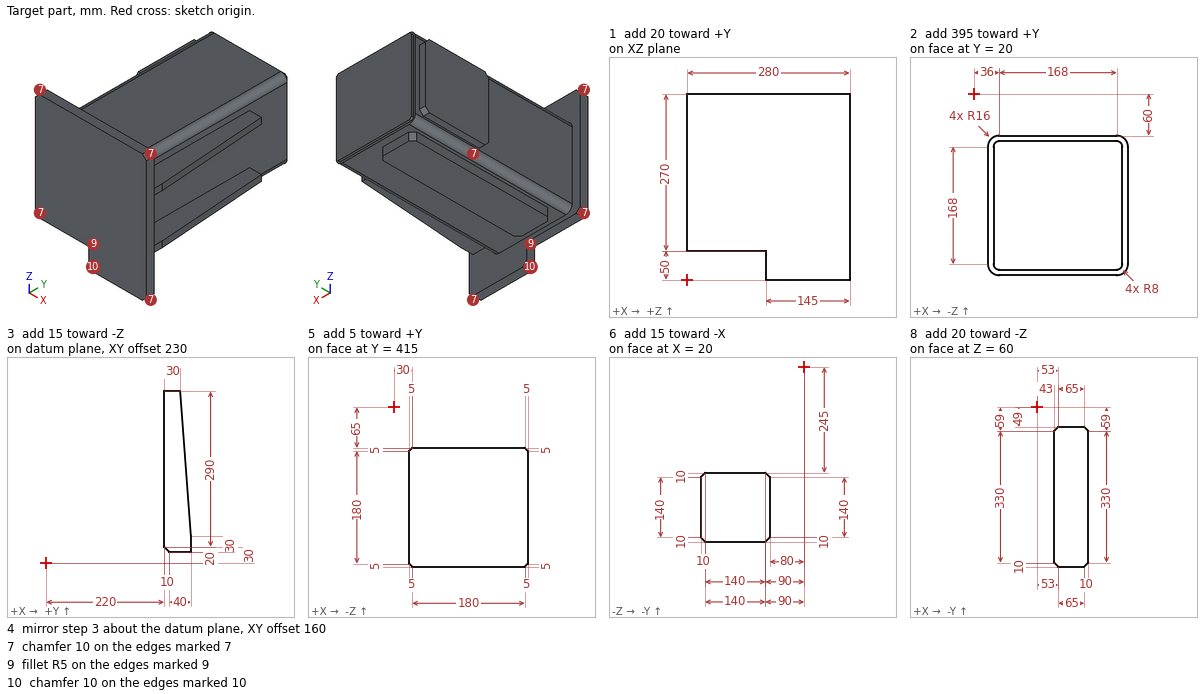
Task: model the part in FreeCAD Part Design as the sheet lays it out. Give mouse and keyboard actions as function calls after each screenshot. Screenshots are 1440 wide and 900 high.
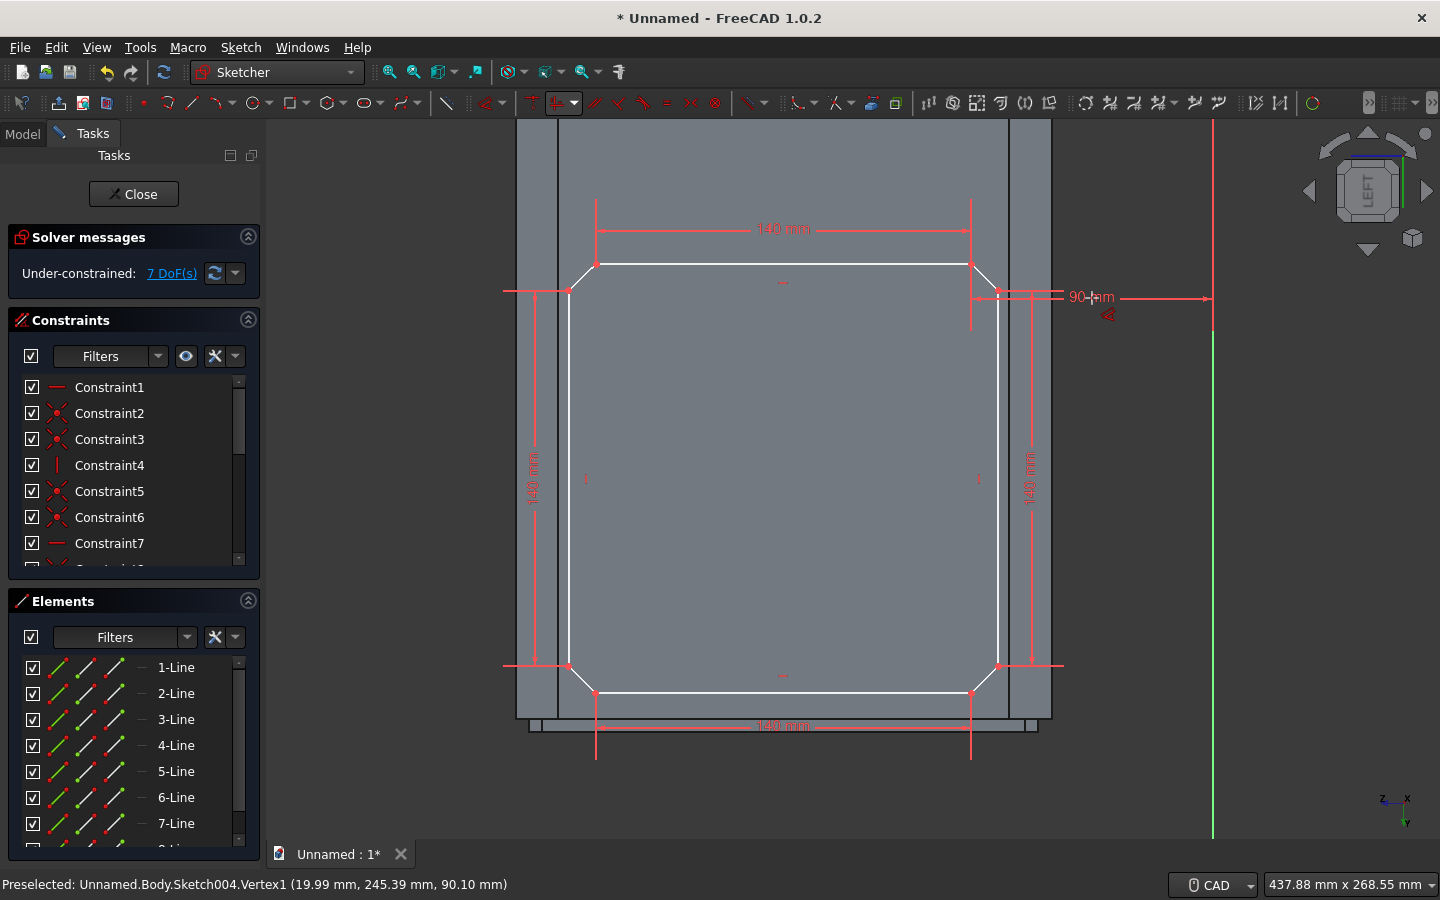
click(971, 693)
click(1092, 727)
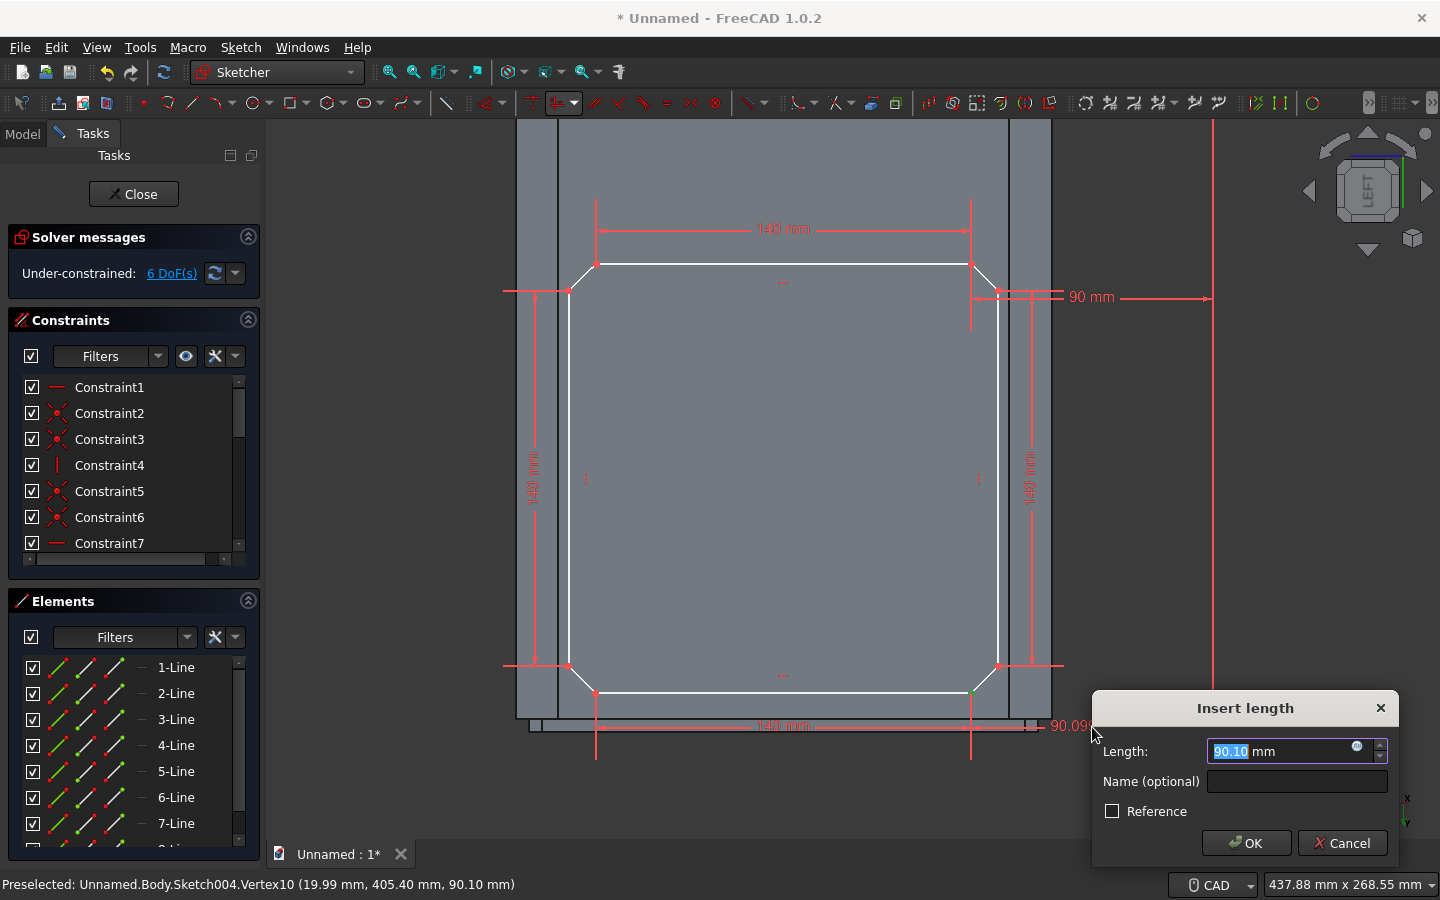
text(90)
key(Return)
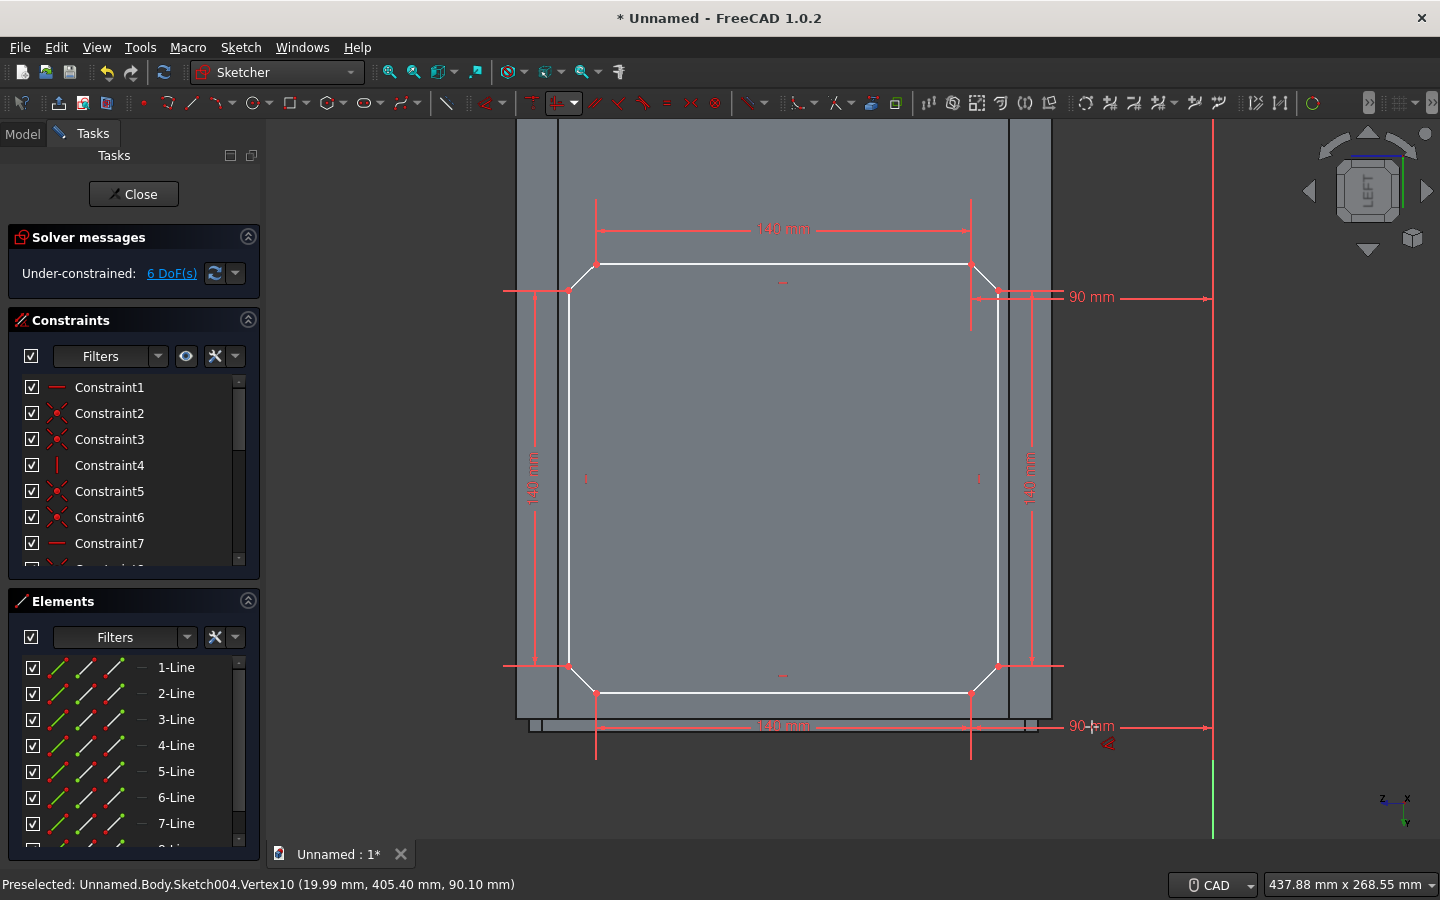
click(998, 666)
click(1105, 700)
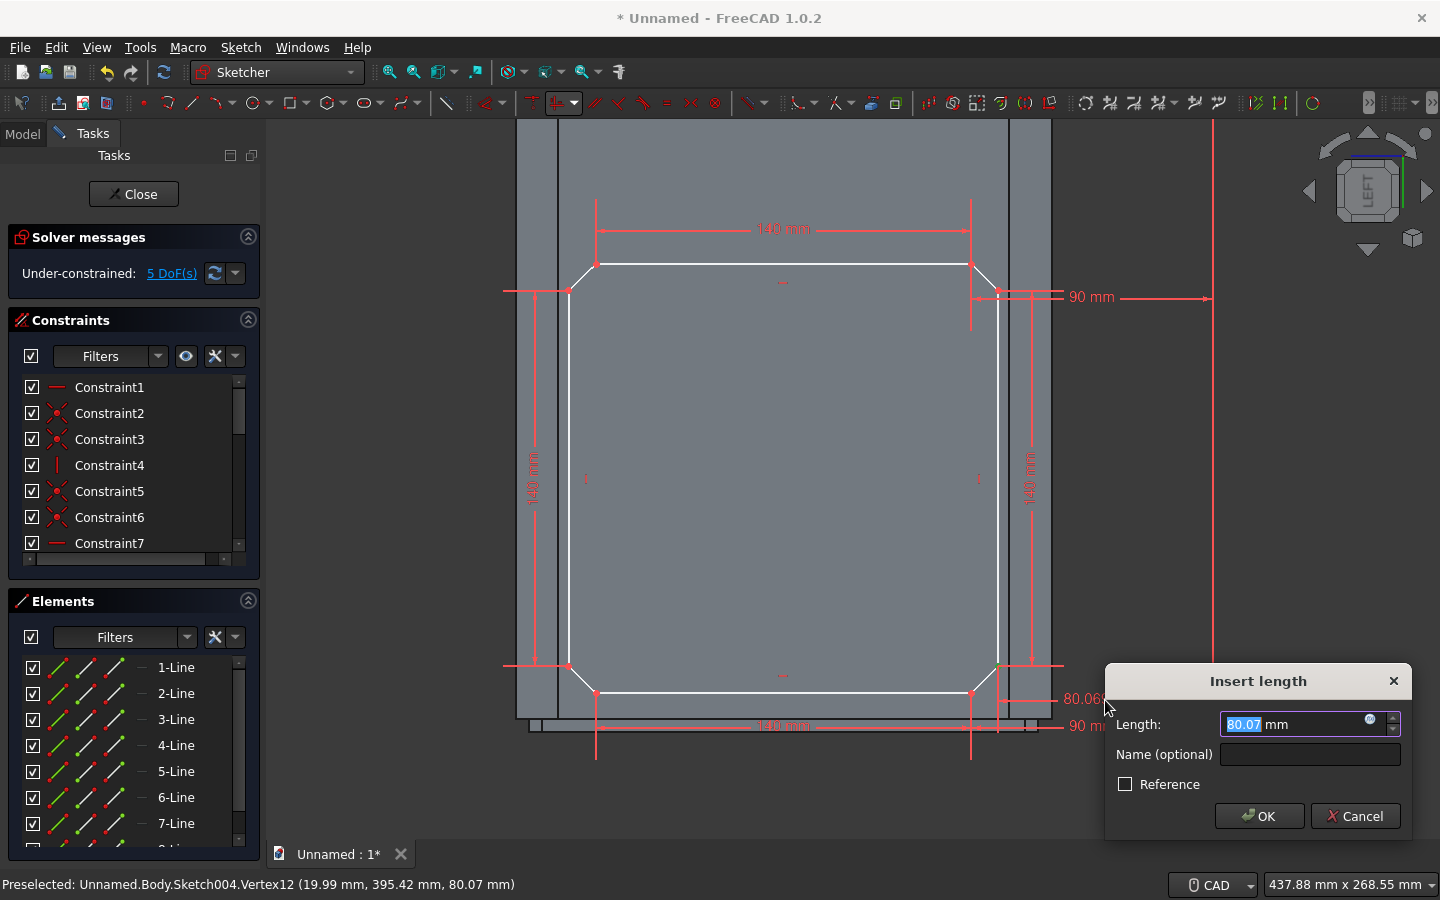
text(80)
key(Return)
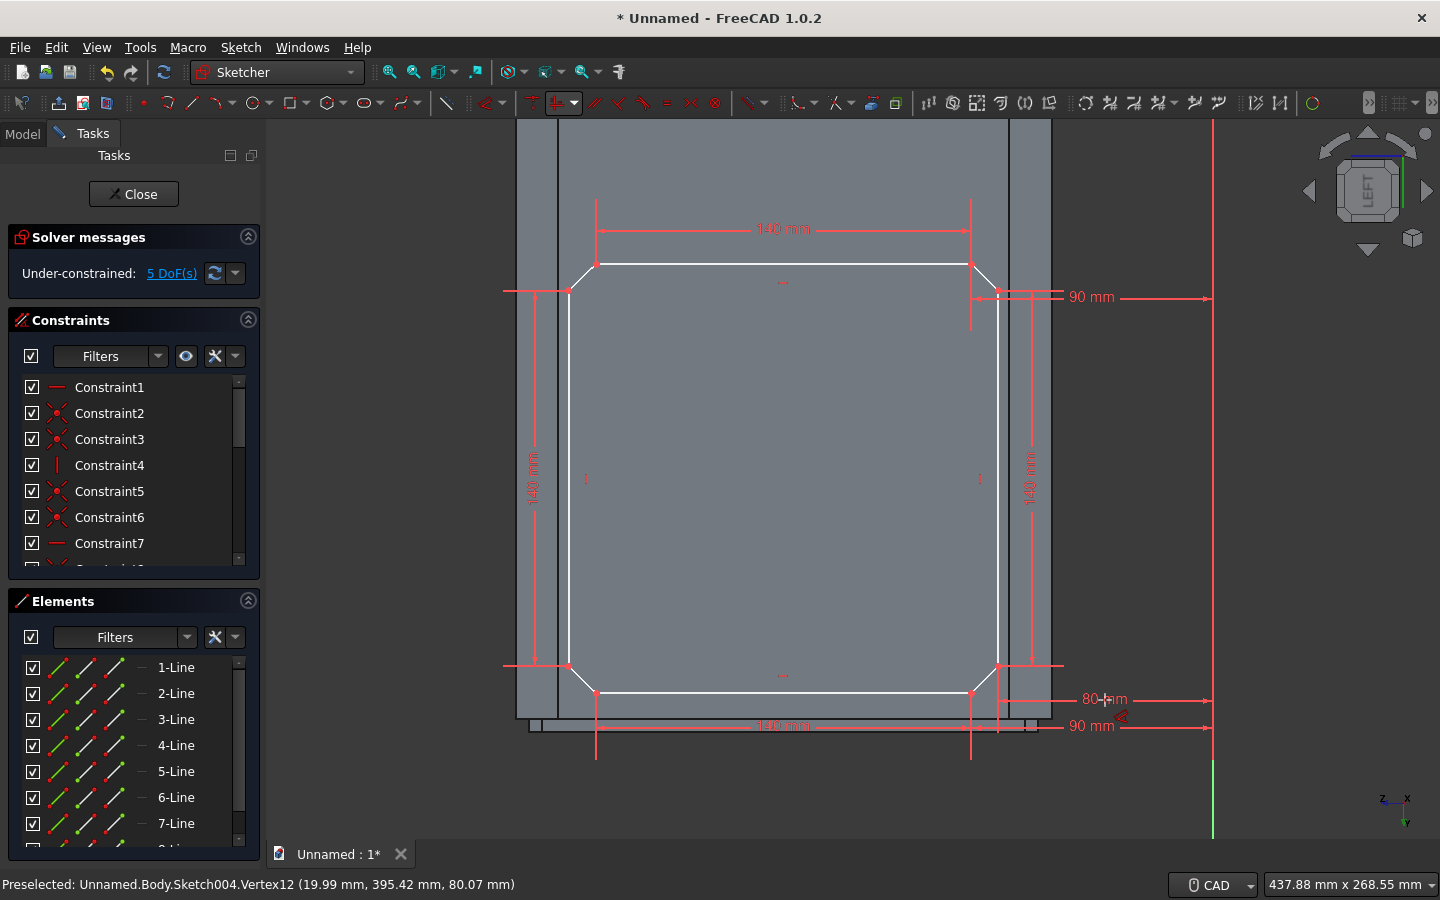
scroll(588, 272, up, 2)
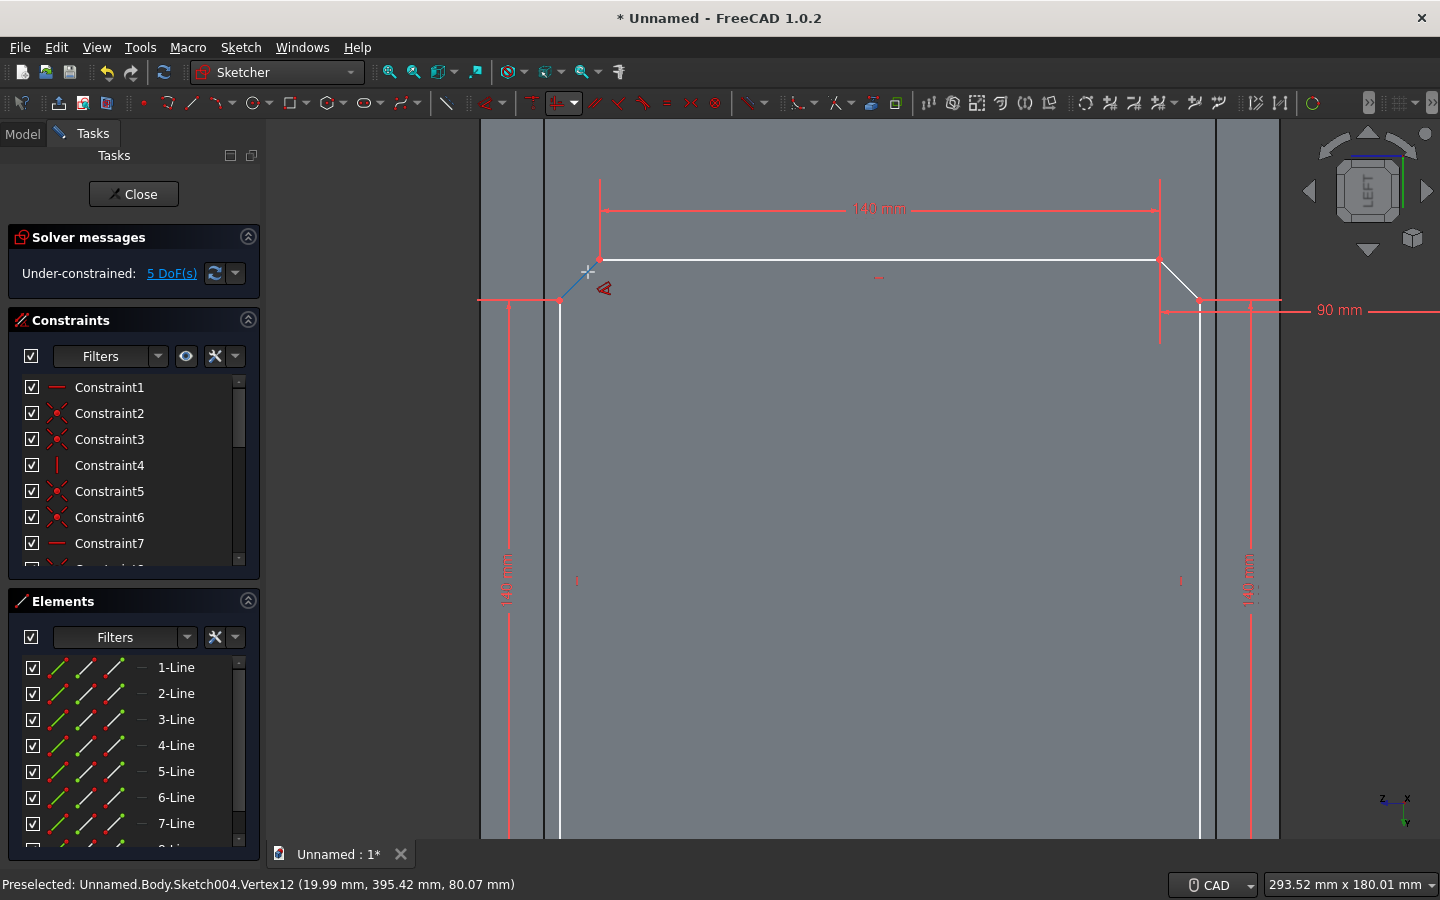
click(588, 272)
click(580, 226)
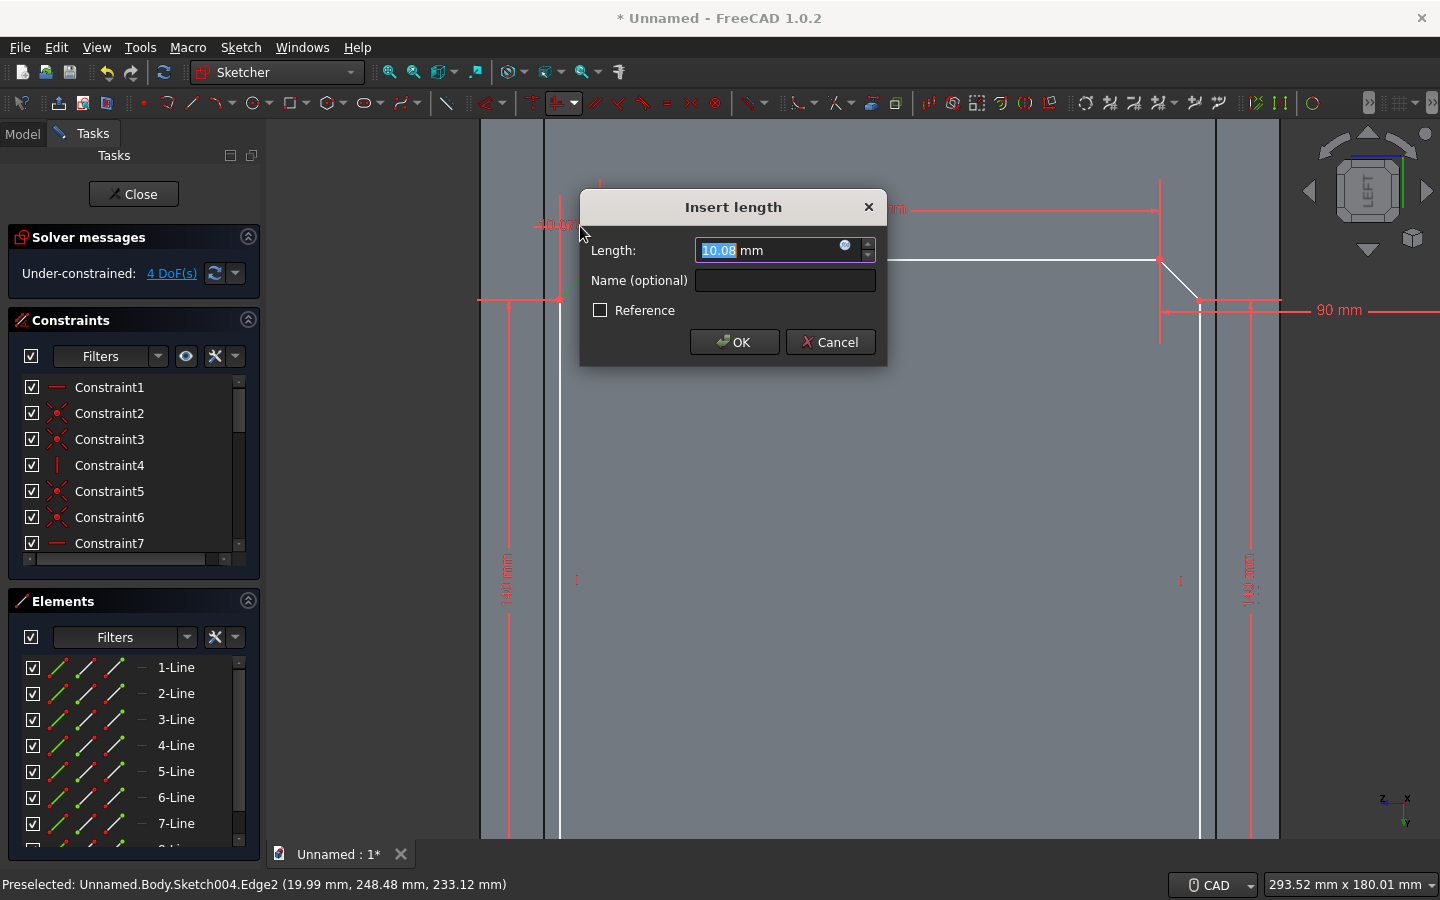
text(10)
key(Return)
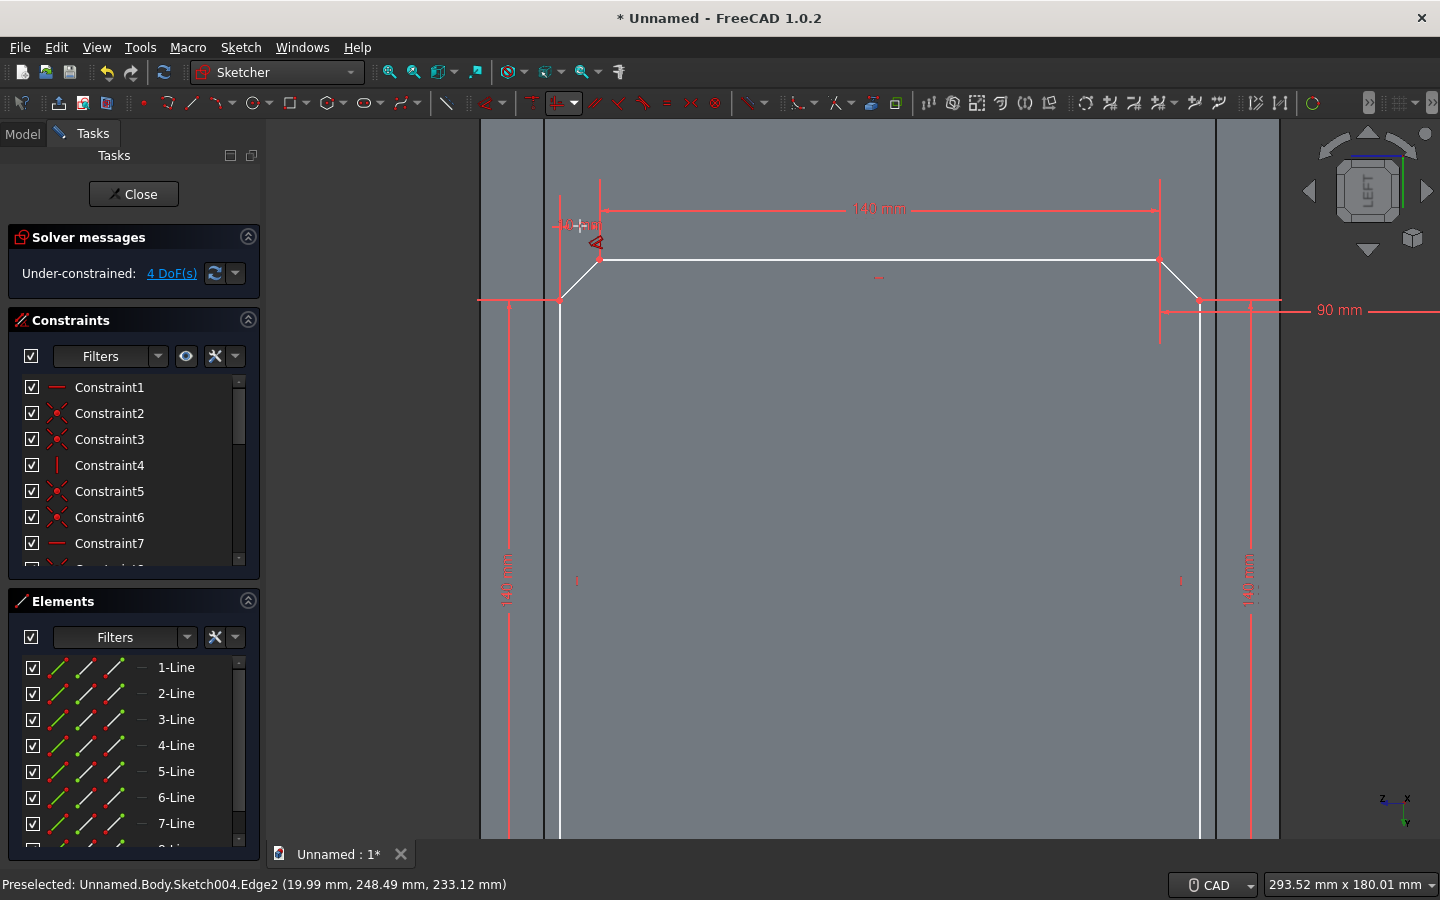
click(588, 272)
click(526, 280)